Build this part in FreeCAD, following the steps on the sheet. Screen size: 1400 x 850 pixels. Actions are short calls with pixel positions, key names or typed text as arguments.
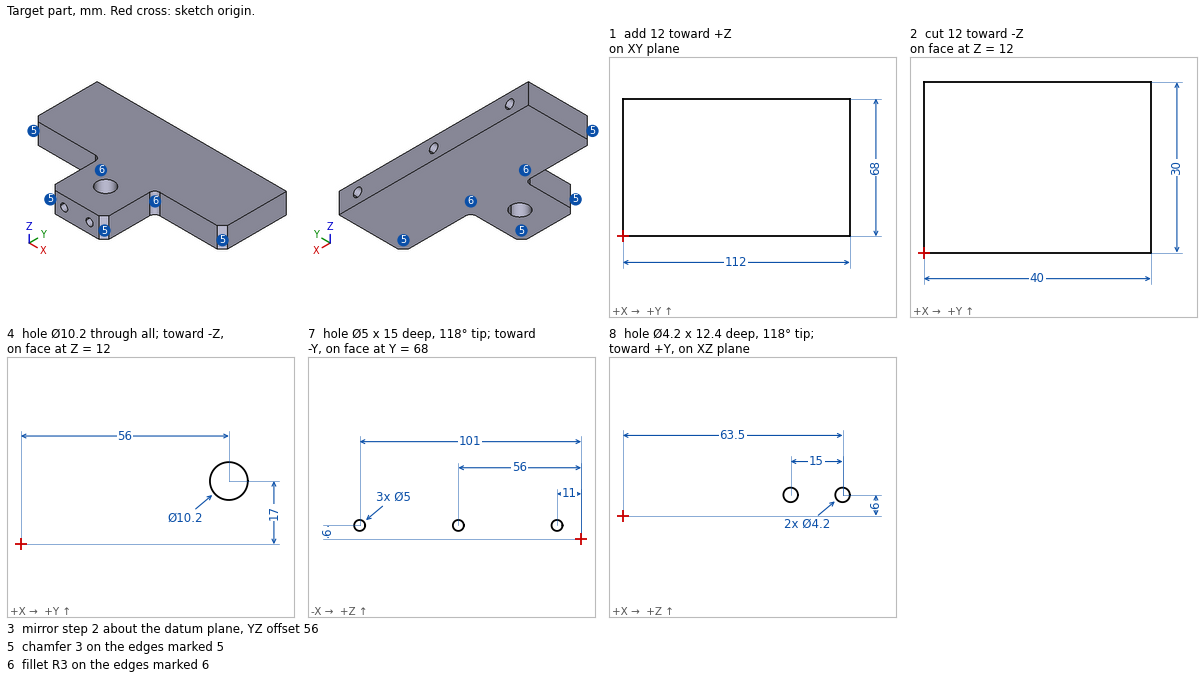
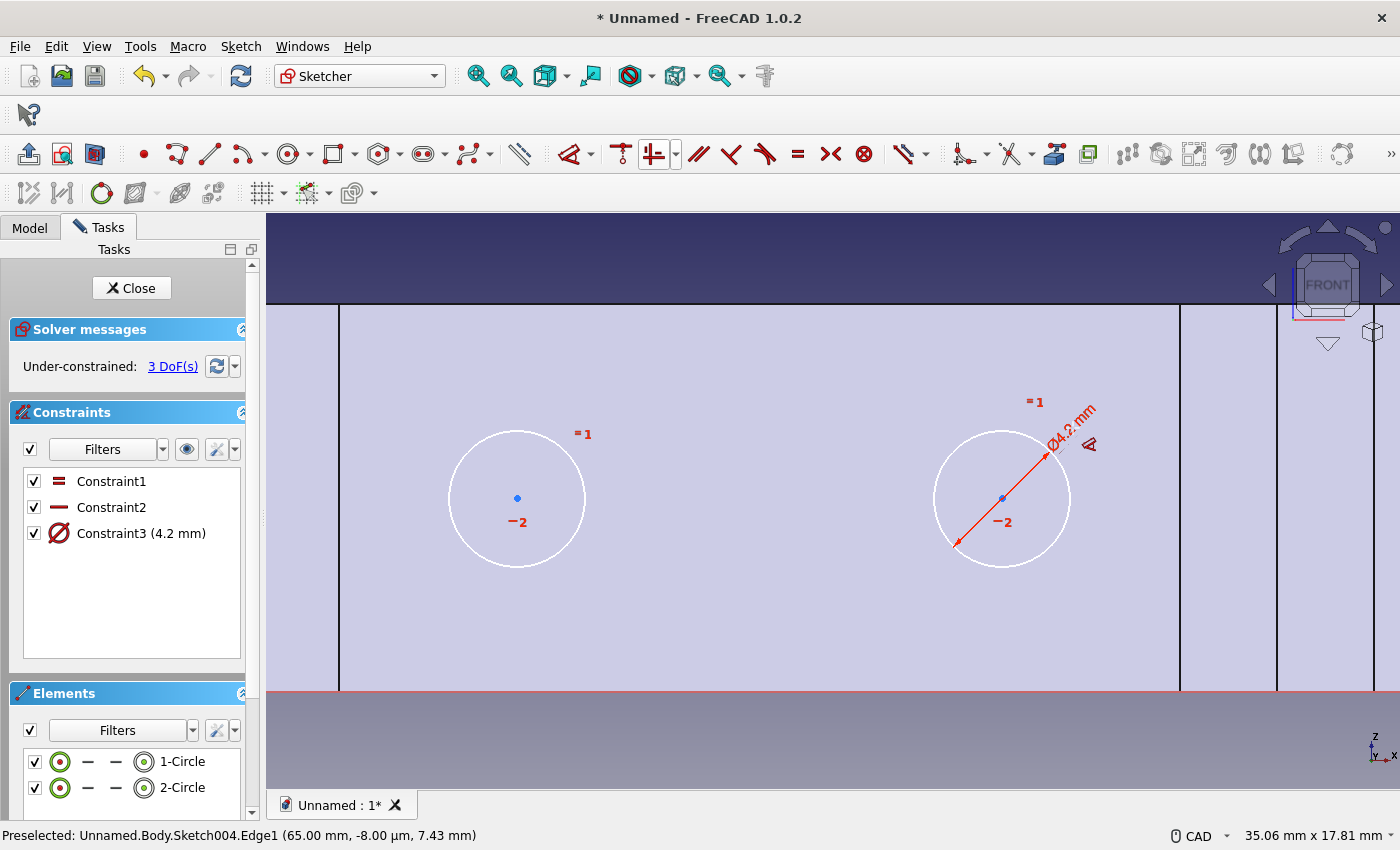
click(1002, 499)
click(1036, 595)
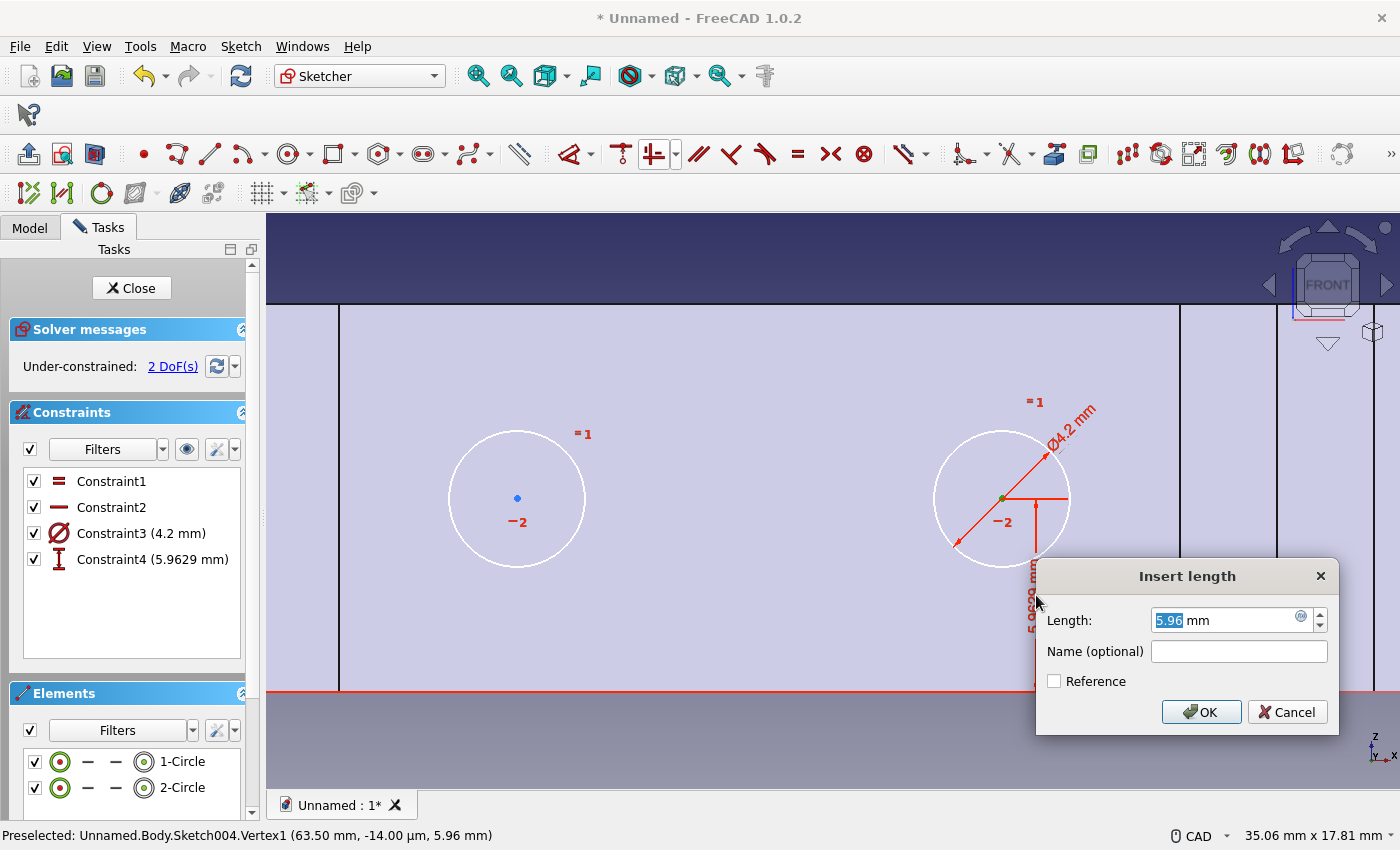
text(6)
key(Return)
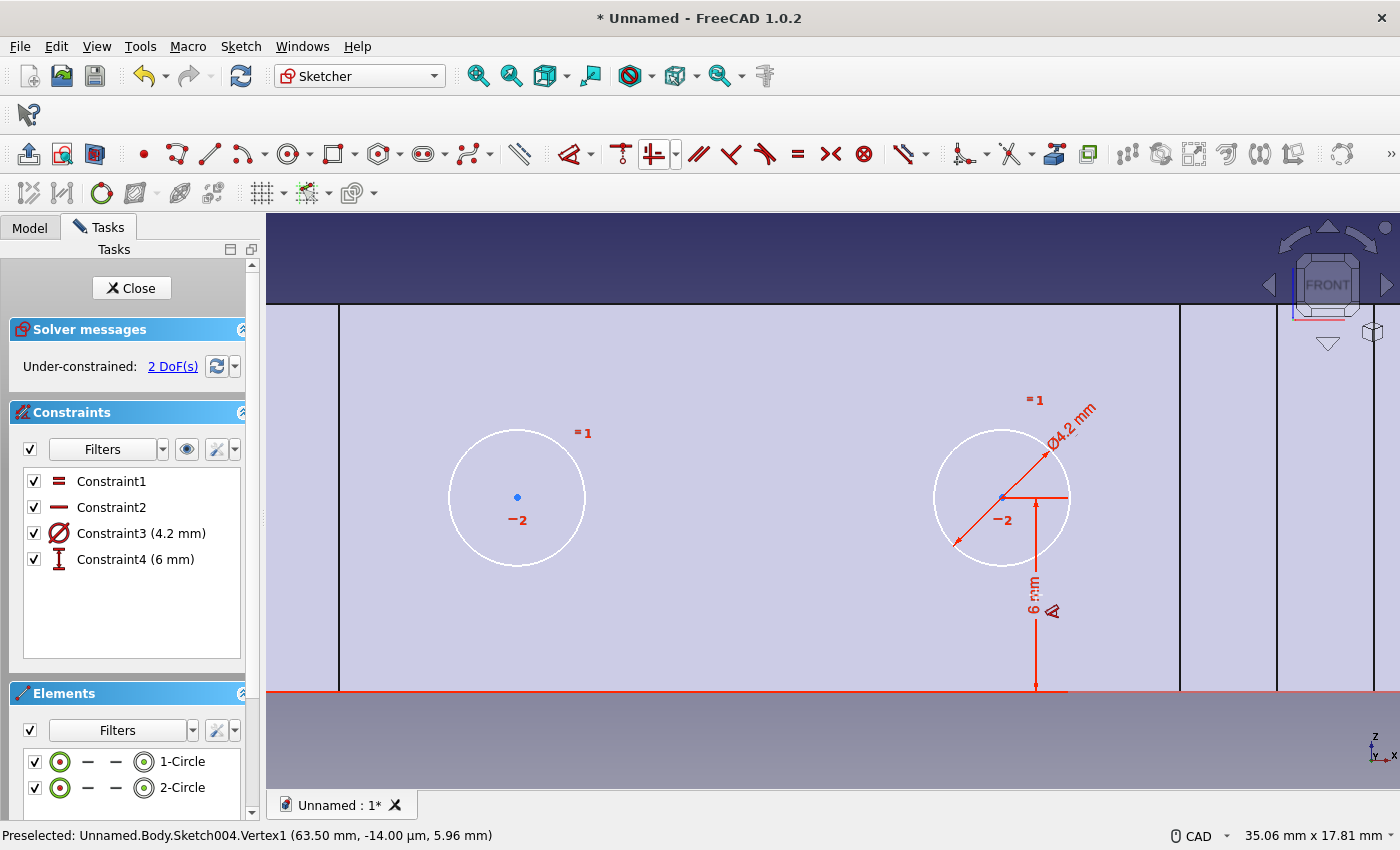
click(1002, 498)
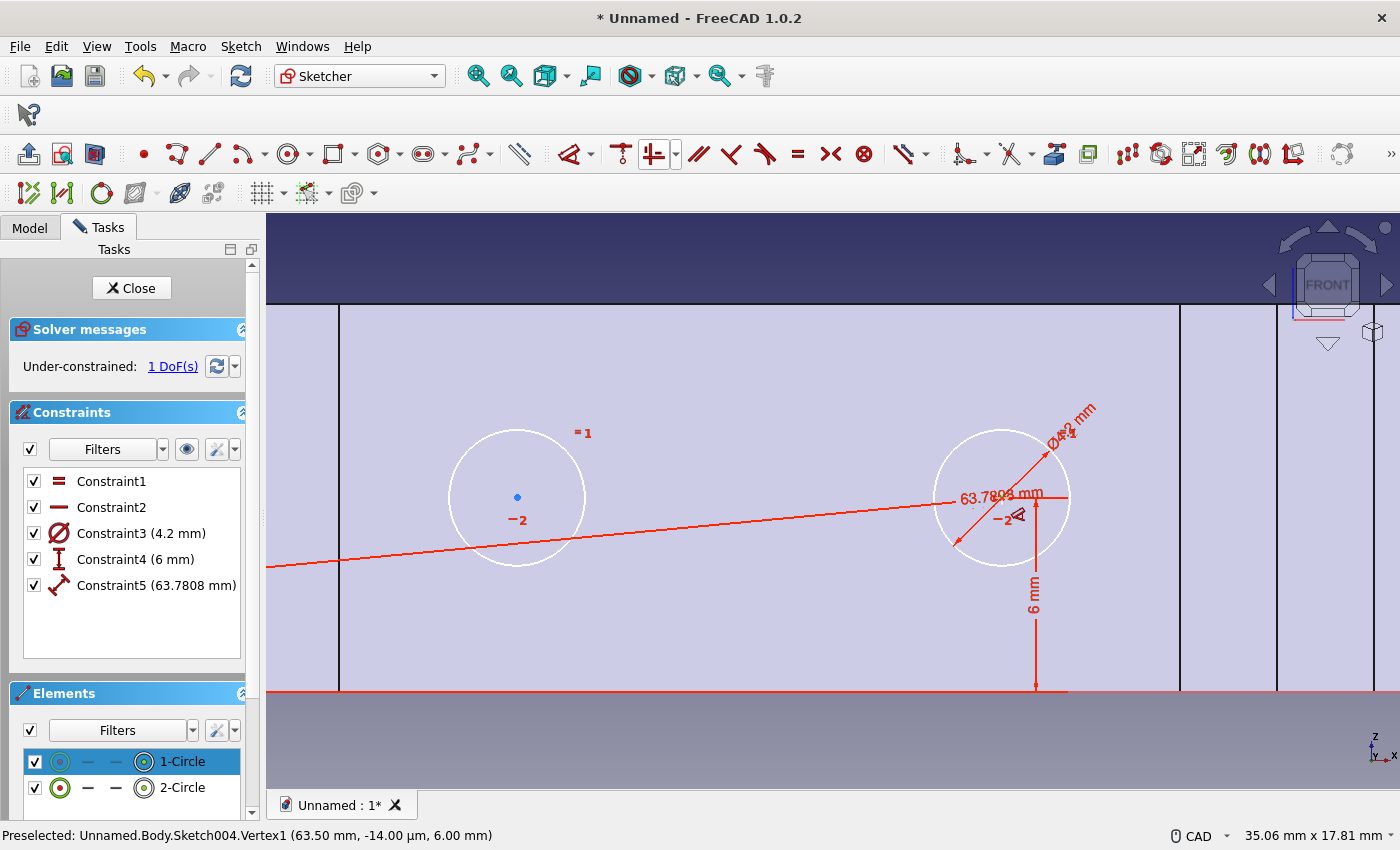
click(517, 498)
click(760, 532)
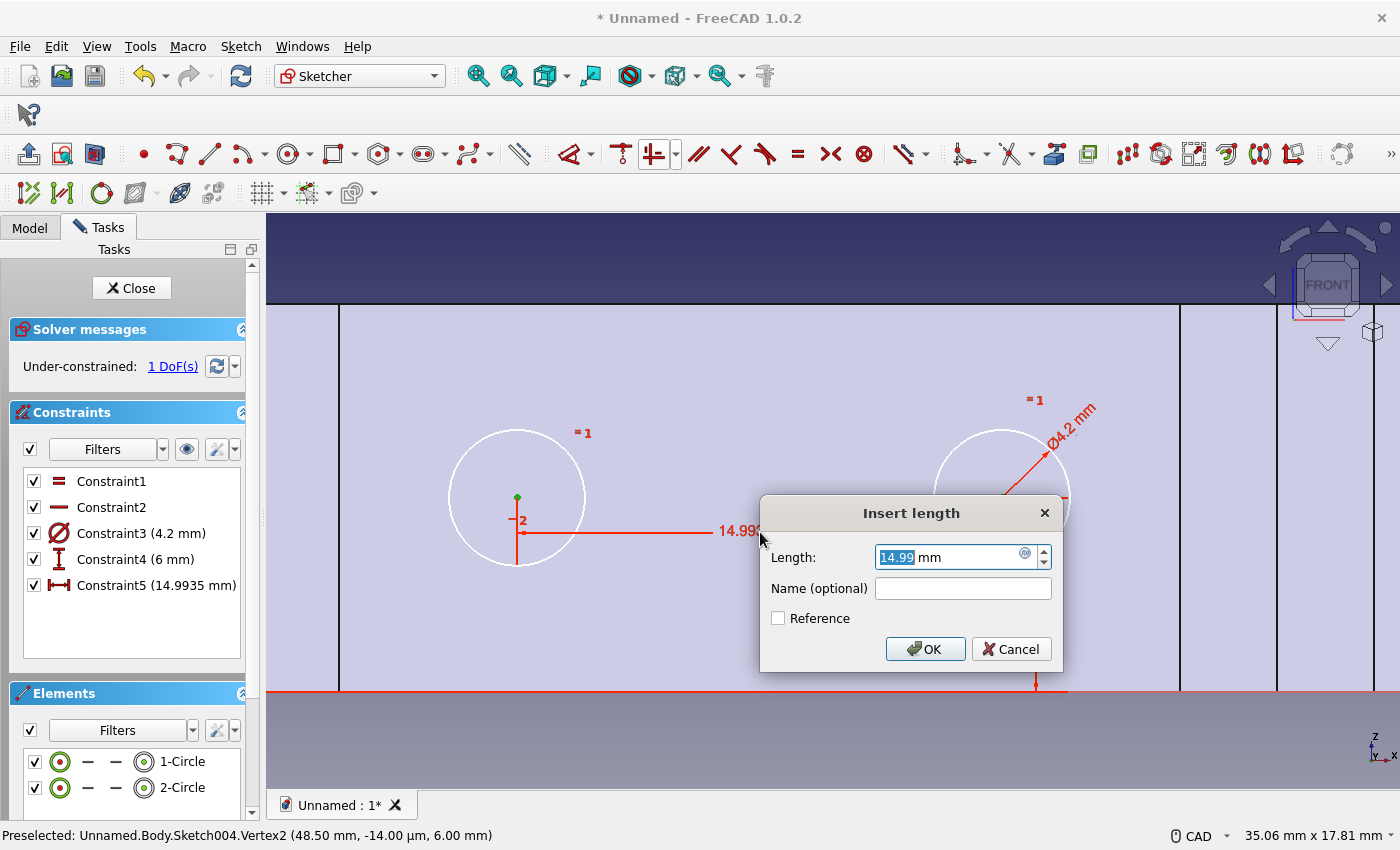
text(15)
key(Return)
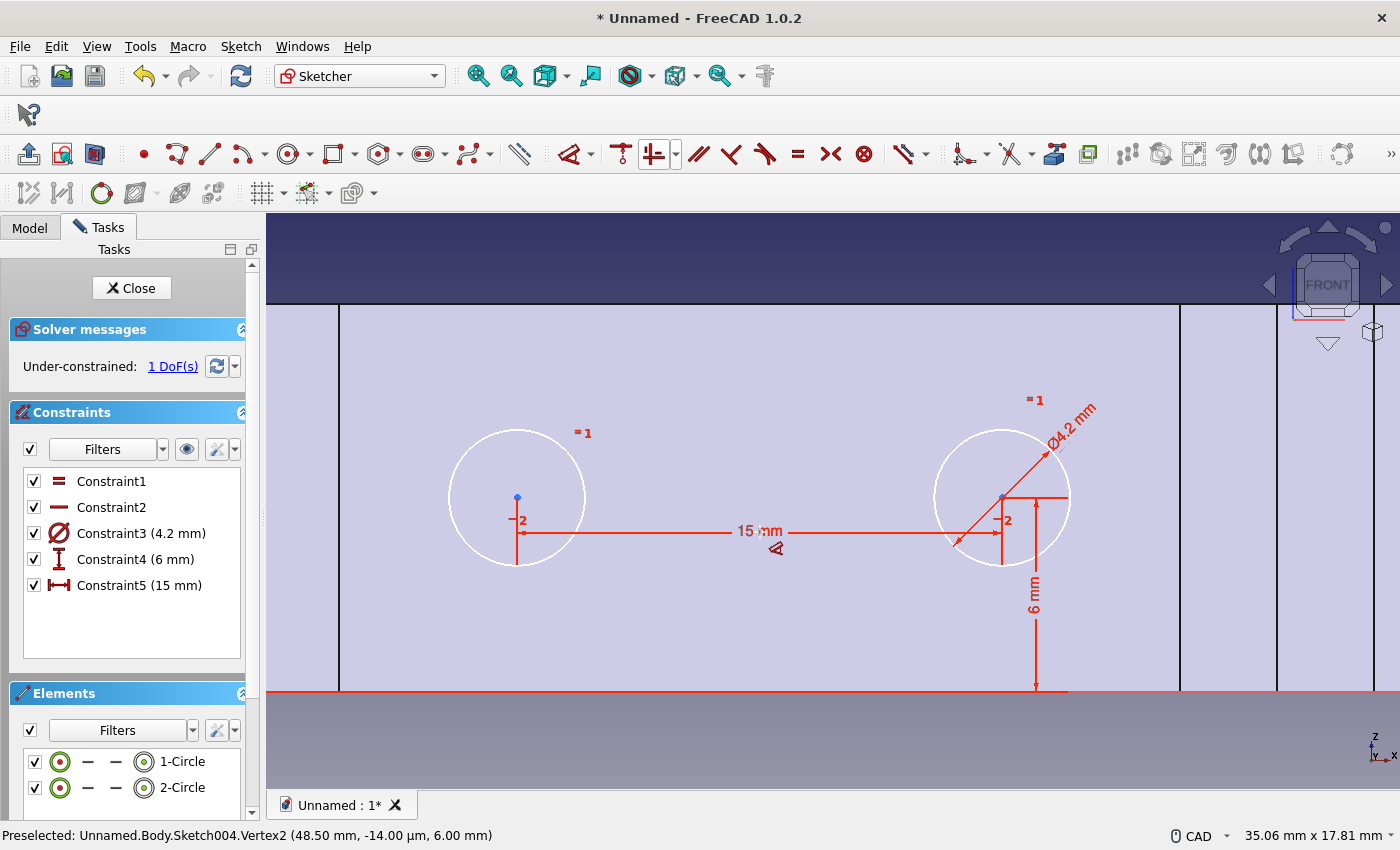
click(1002, 498)
click(648, 726)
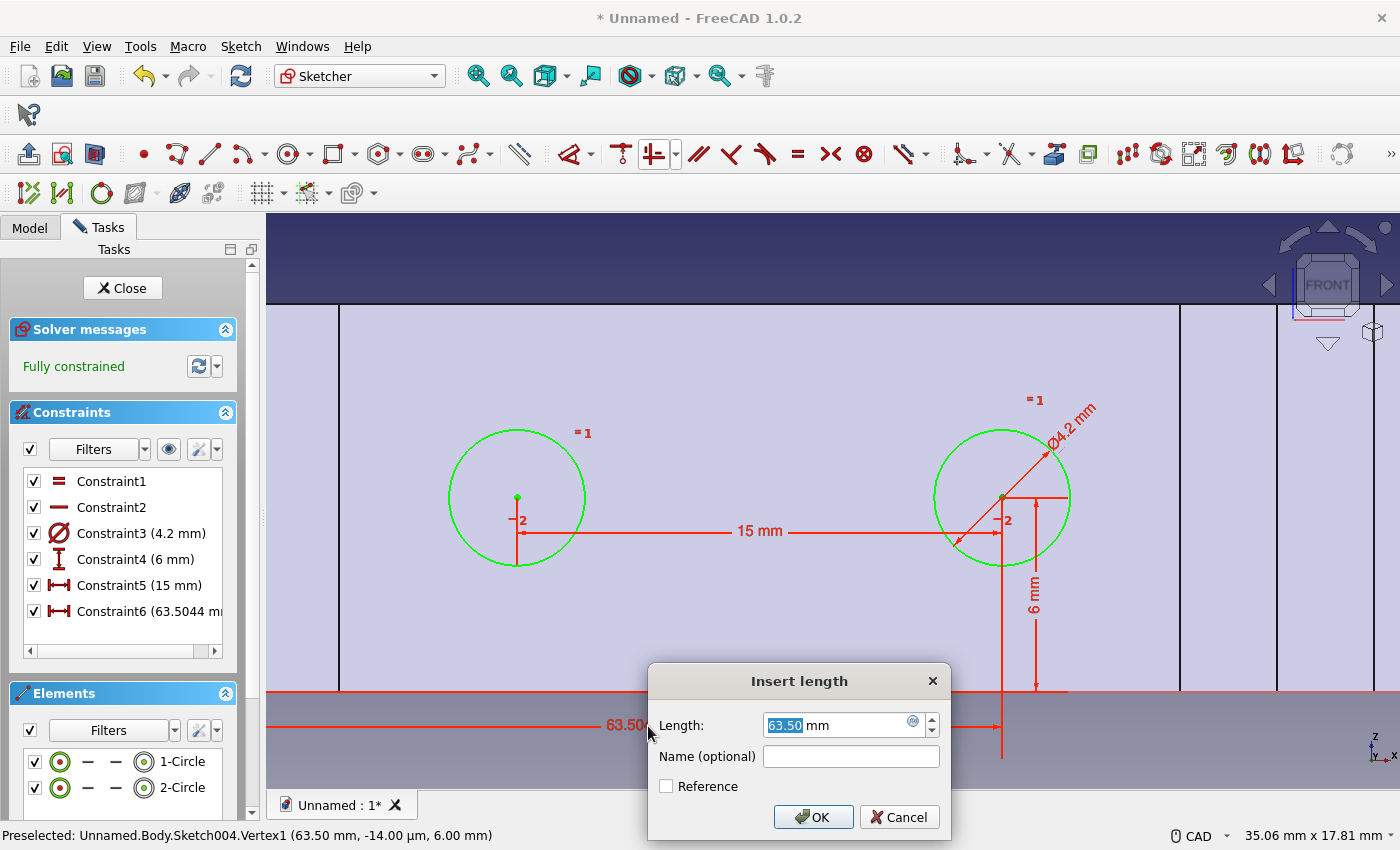
text(63.5)
key(Return)
key(Escape)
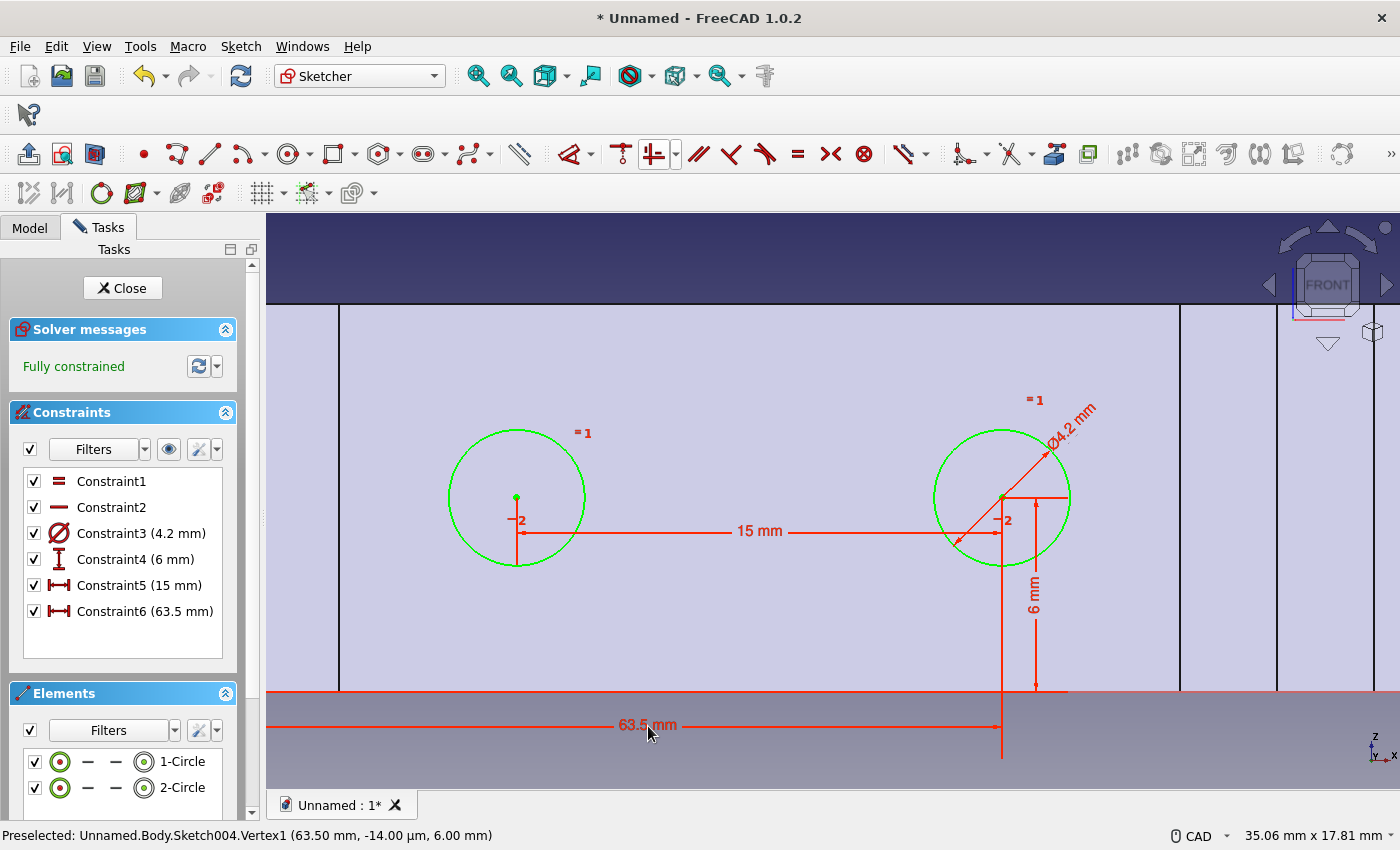
click(123, 288)